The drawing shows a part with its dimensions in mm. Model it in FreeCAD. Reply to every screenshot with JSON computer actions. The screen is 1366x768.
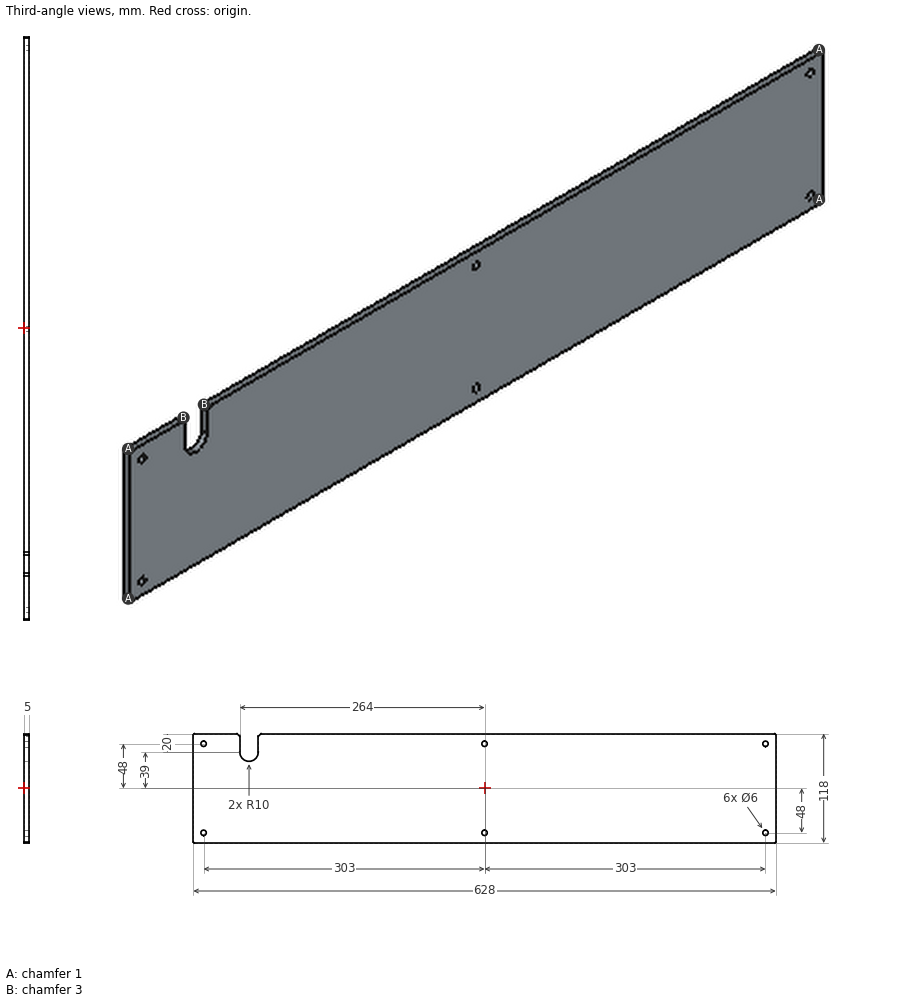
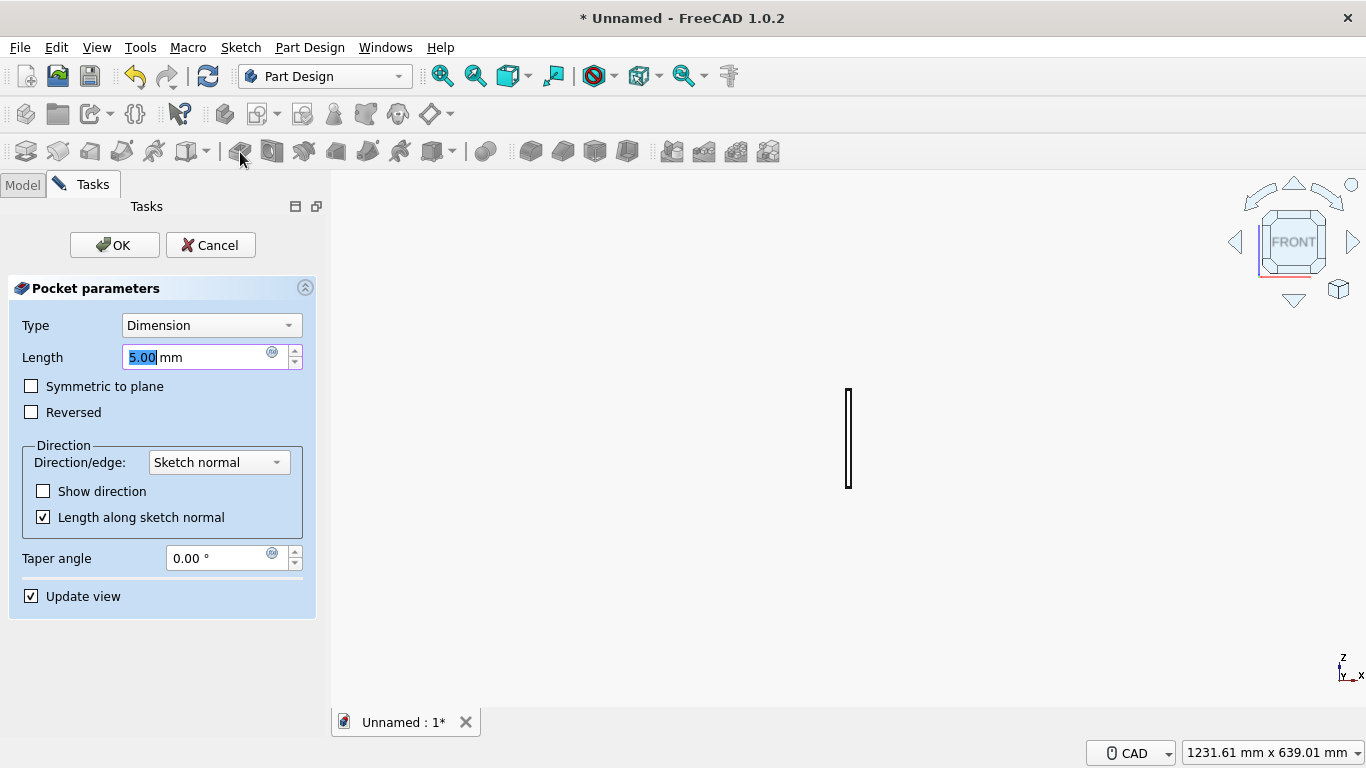
{"action": "left_click", "coordinate": [212, 326]}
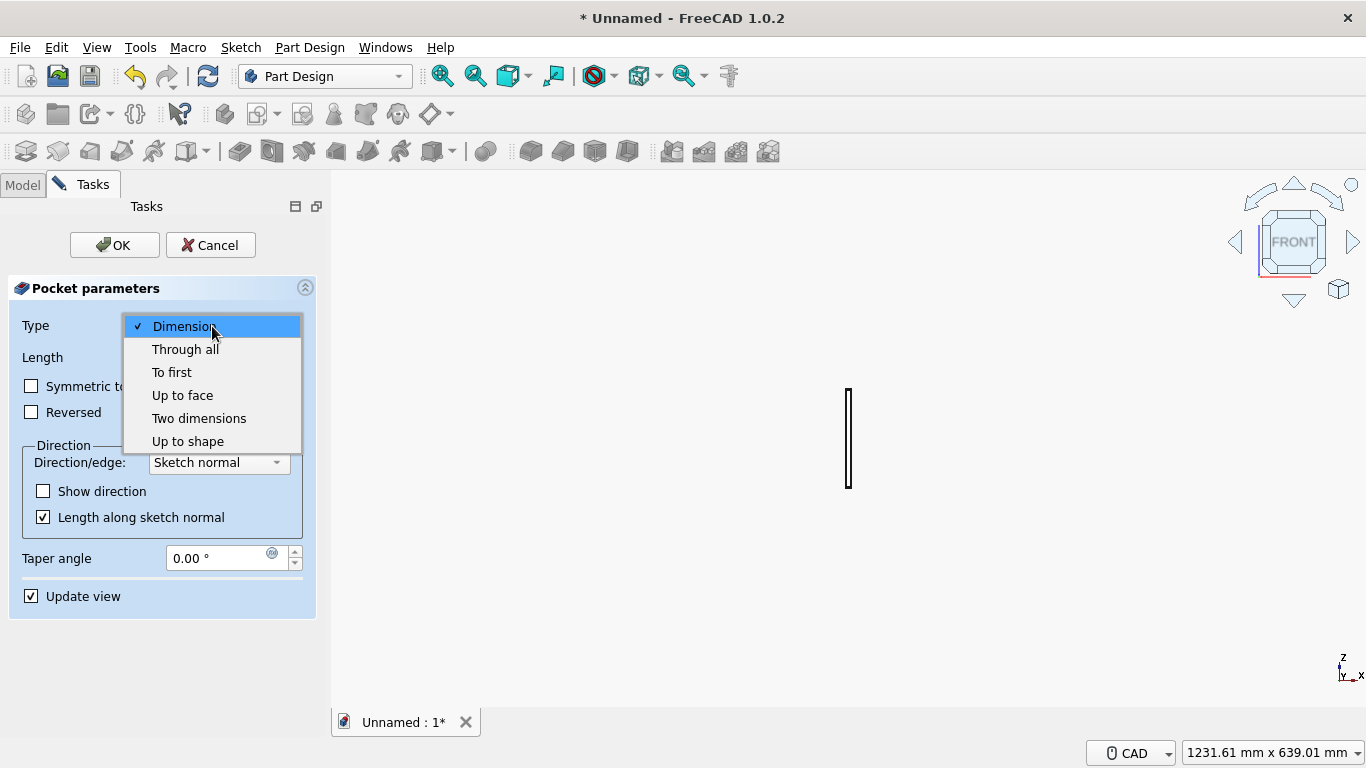
{"action": "left_click", "coordinate": [212, 350]}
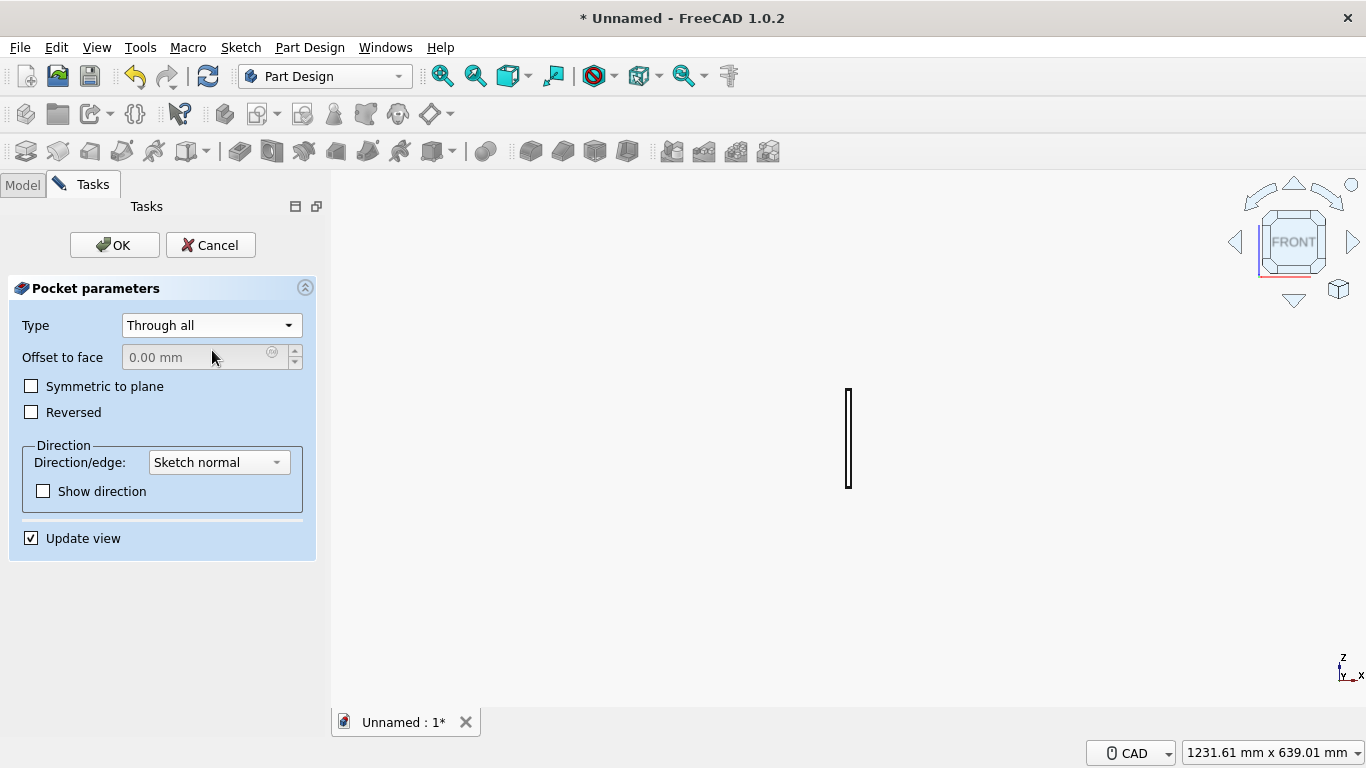
{"action": "left_click", "coordinate": [30, 412]}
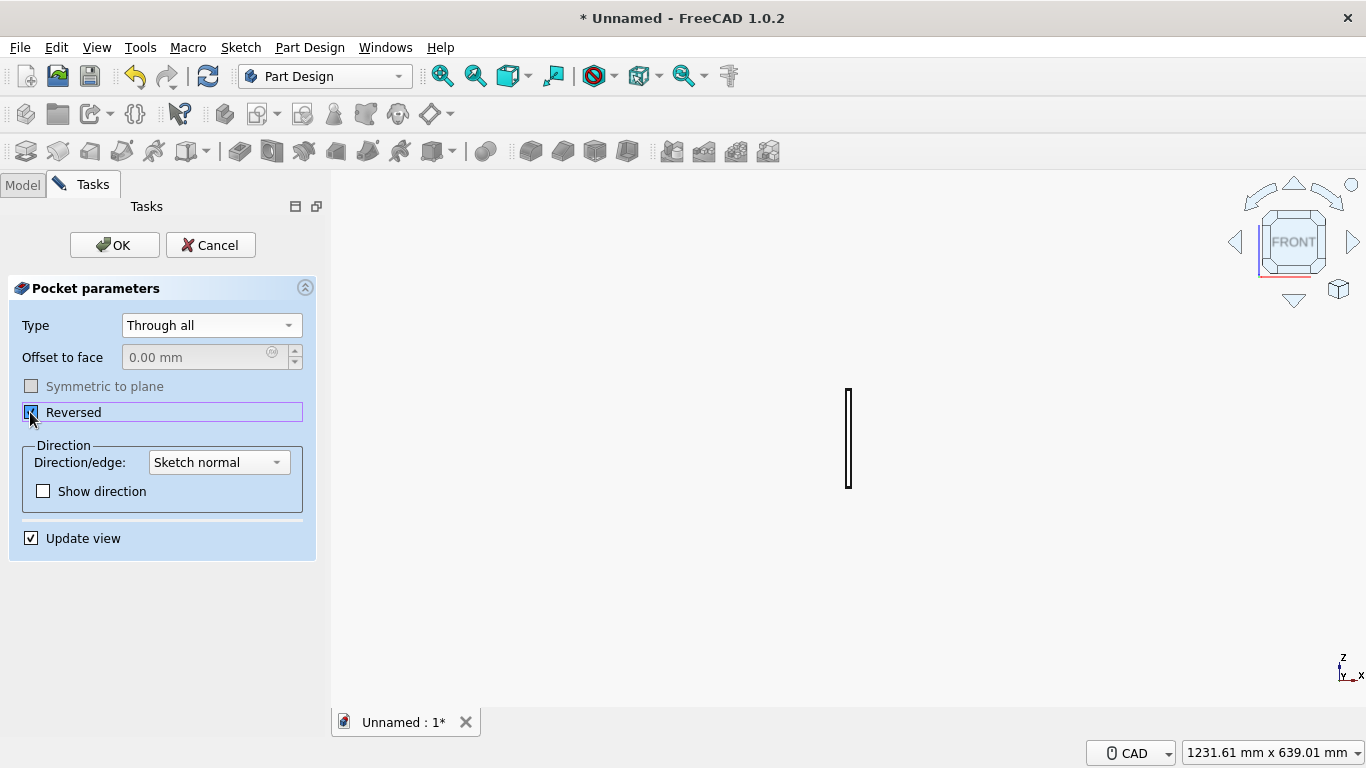
{"action": "left_click", "coordinate": [115, 245]}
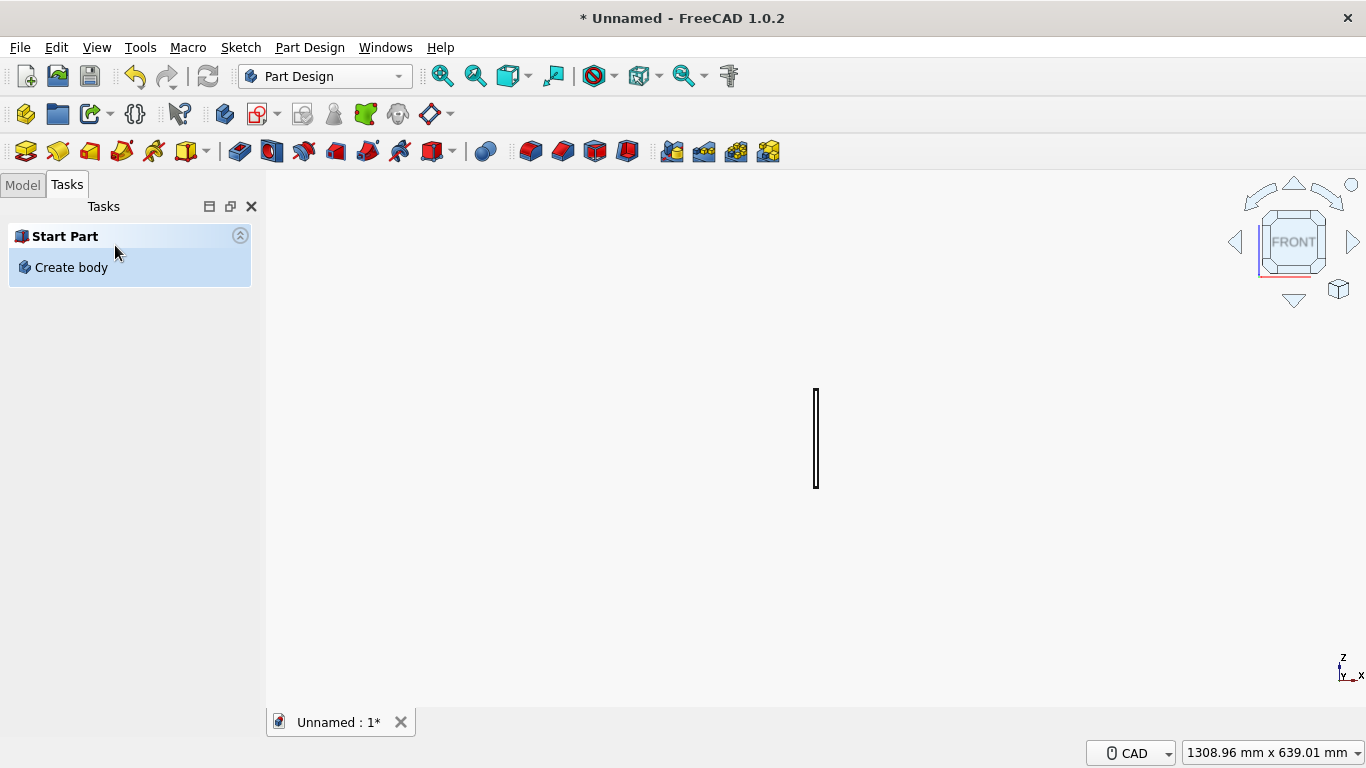
{"action": "left_click", "coordinate": [444, 76]}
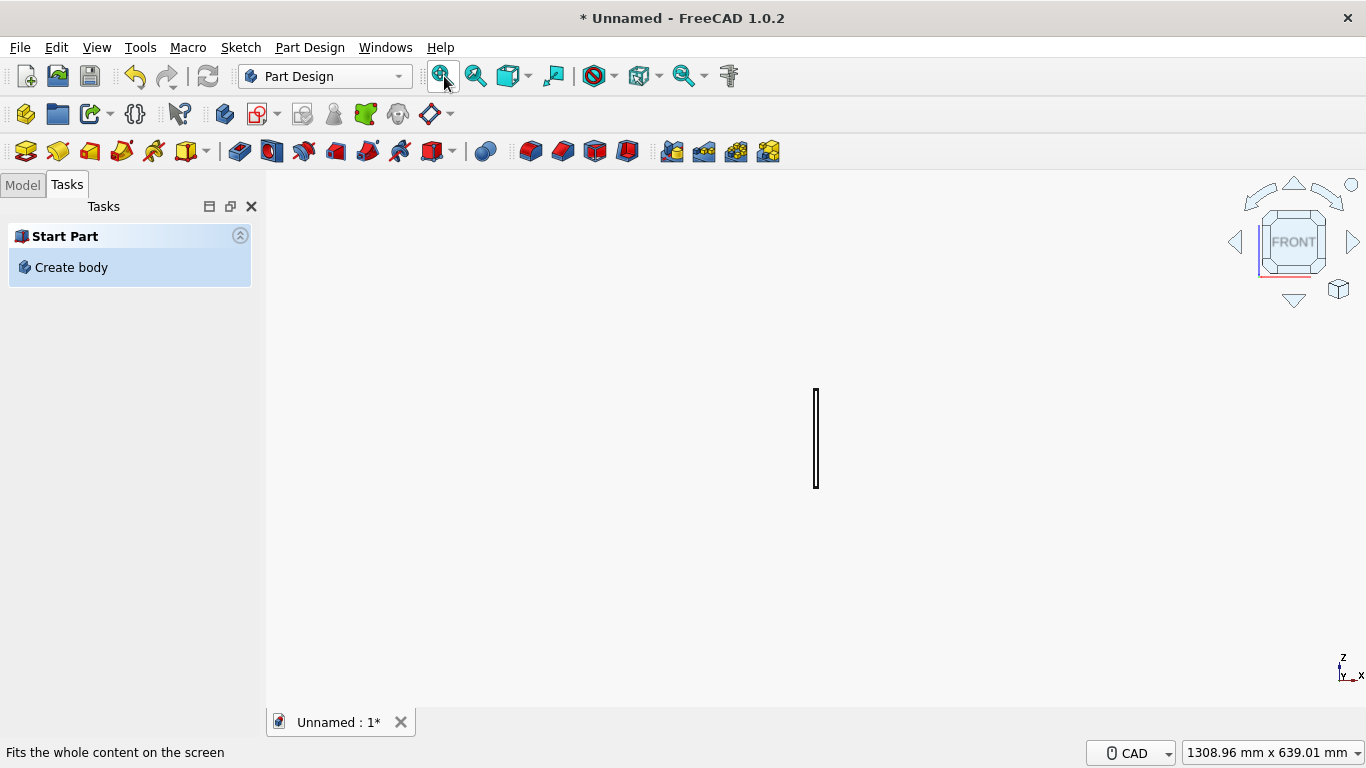
{"action": "key", "text": "0"}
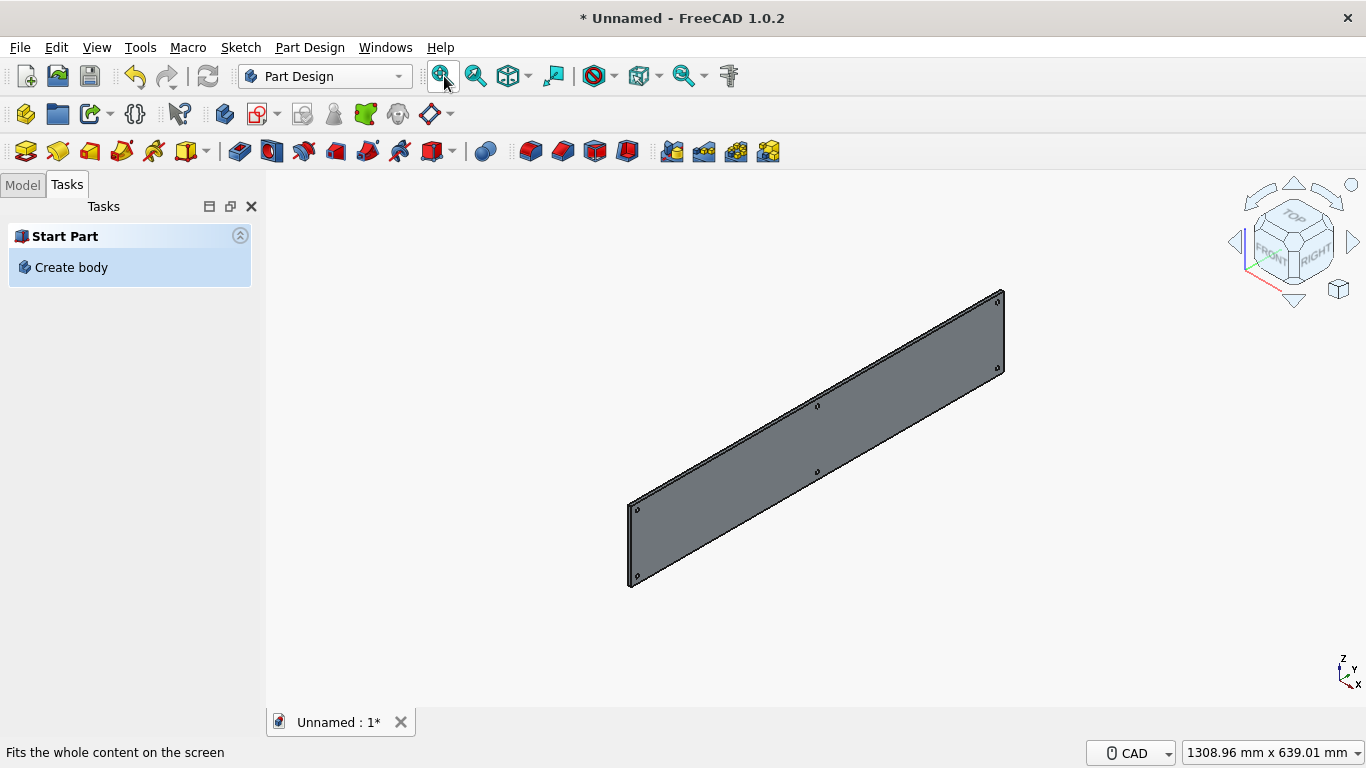
{"action": "left_click", "coordinate": [924, 377]}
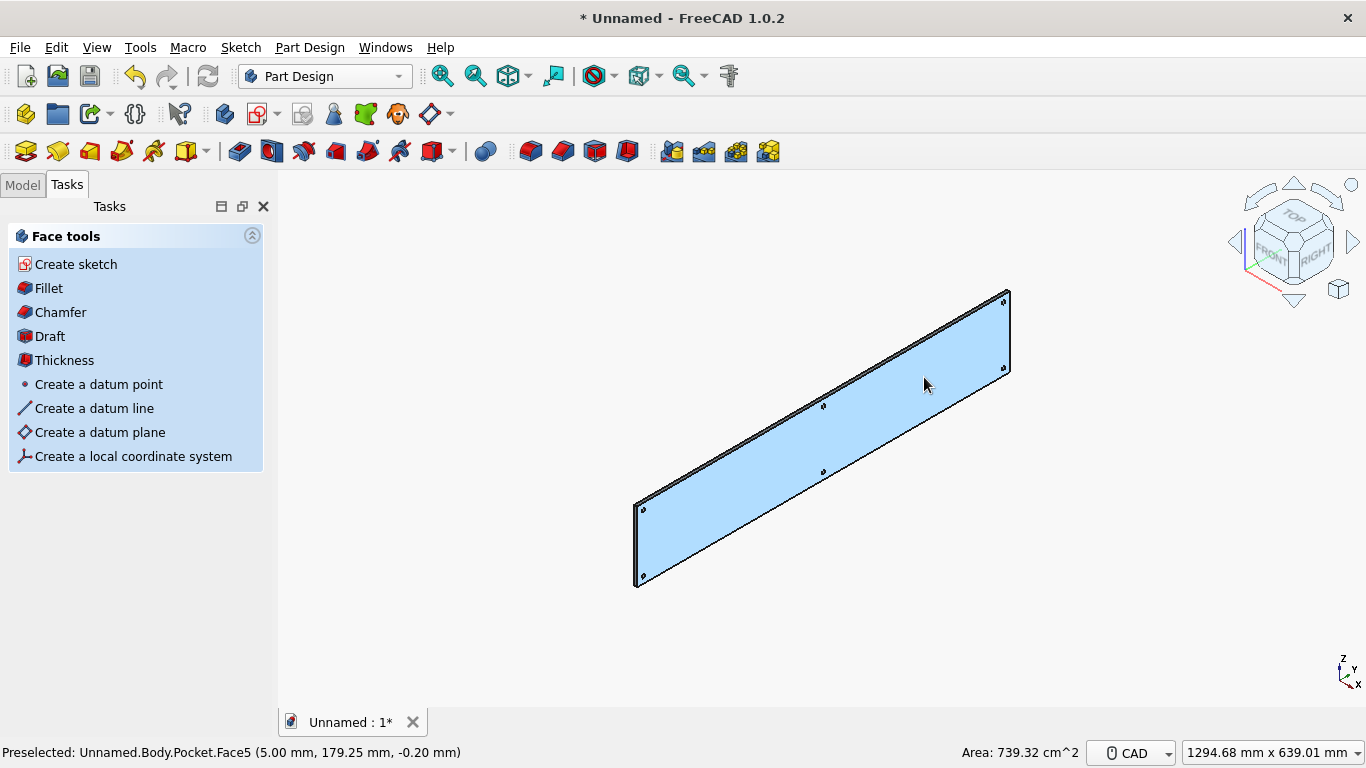
{"action": "left_click", "coordinate": [258, 114]}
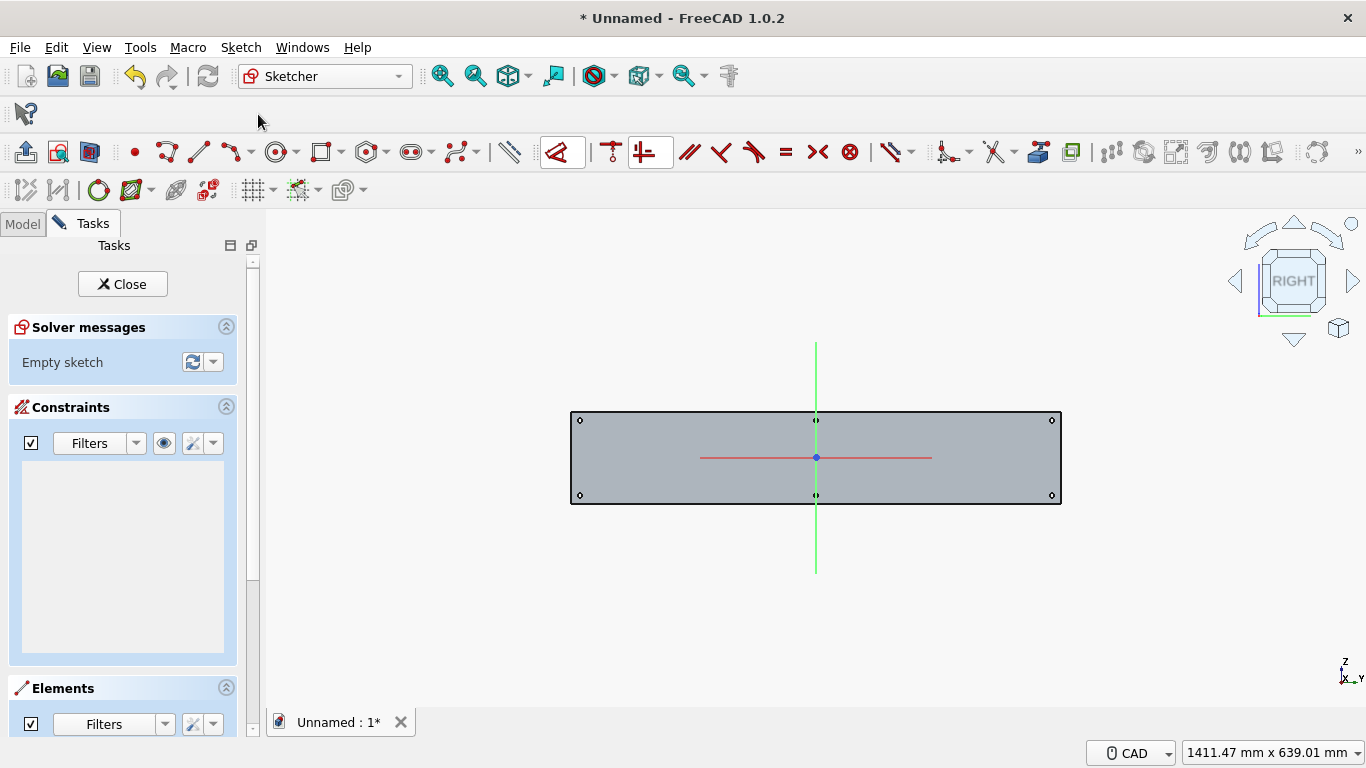
{"action": "scroll", "coordinate": [605, 416], "scroll_direction": "up", "scroll_amount": 12}